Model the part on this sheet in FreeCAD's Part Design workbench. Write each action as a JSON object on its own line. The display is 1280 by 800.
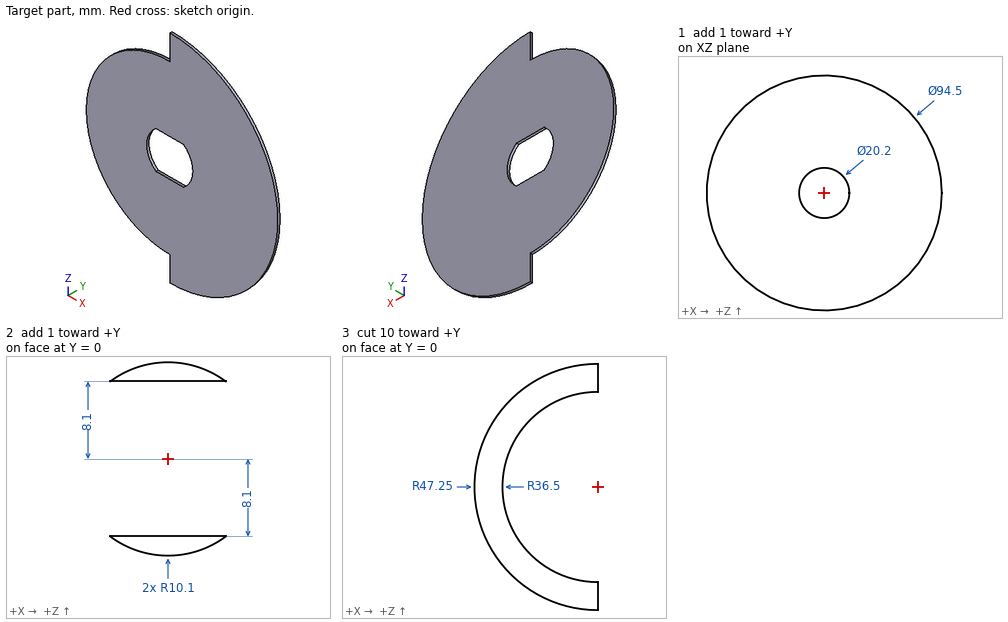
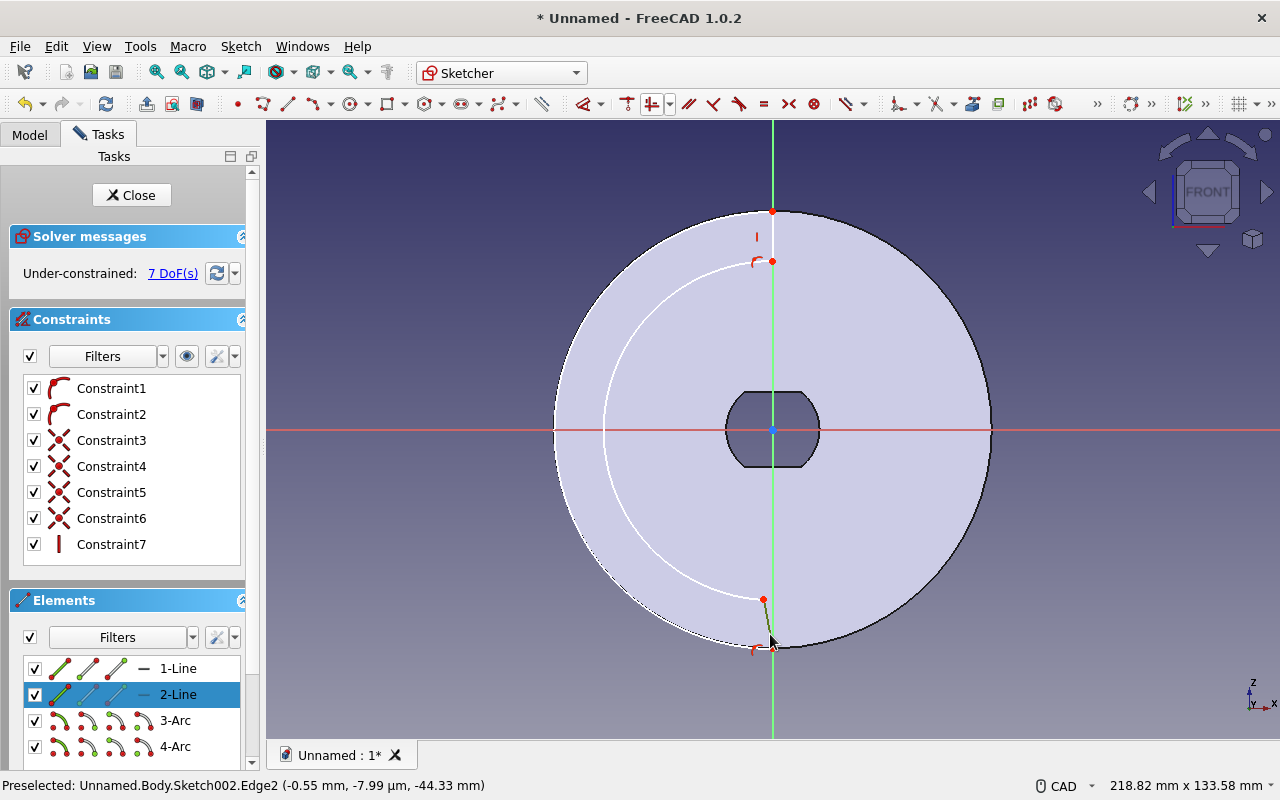
{"action": "left_click", "coordinate": [670, 104]}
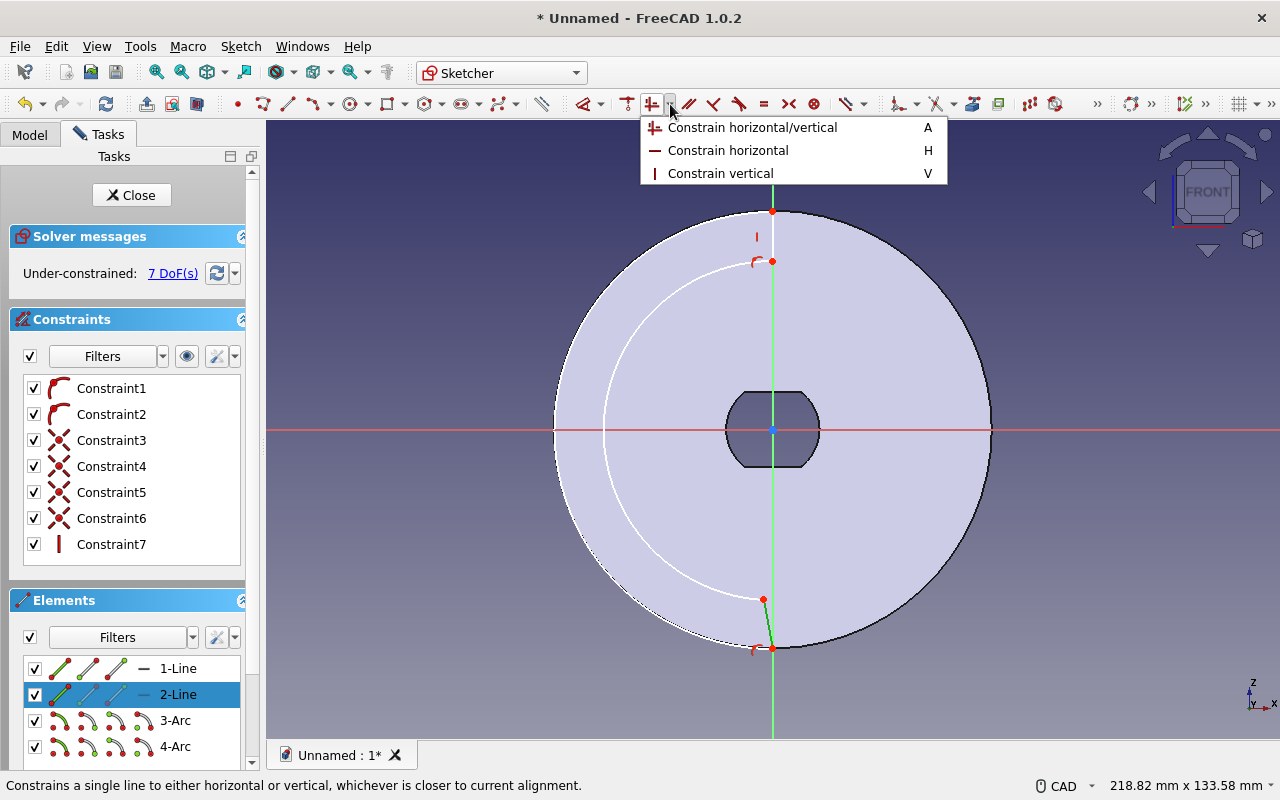
{"action": "left_click", "coordinate": [794, 174]}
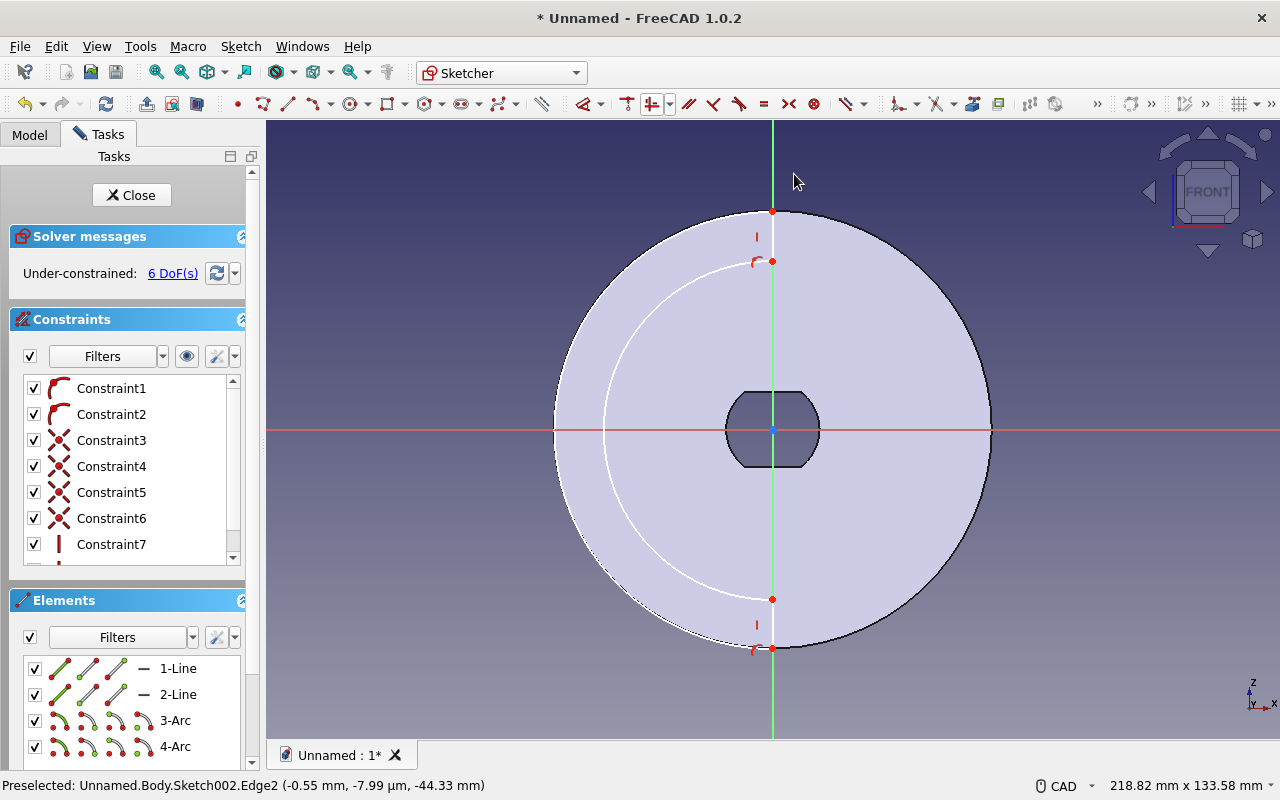
{"action": "left_click", "coordinate": [596, 302]}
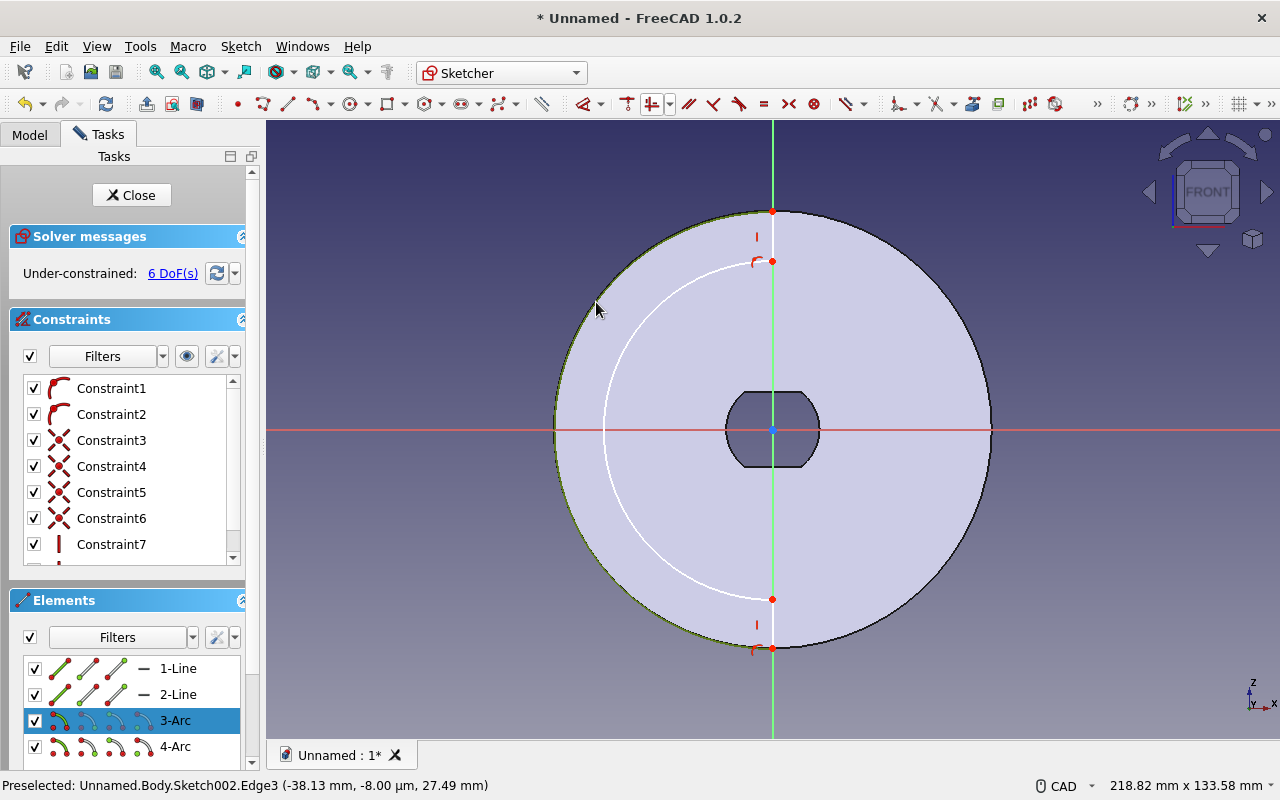
{"action": "left_click", "coordinate": [636, 331]}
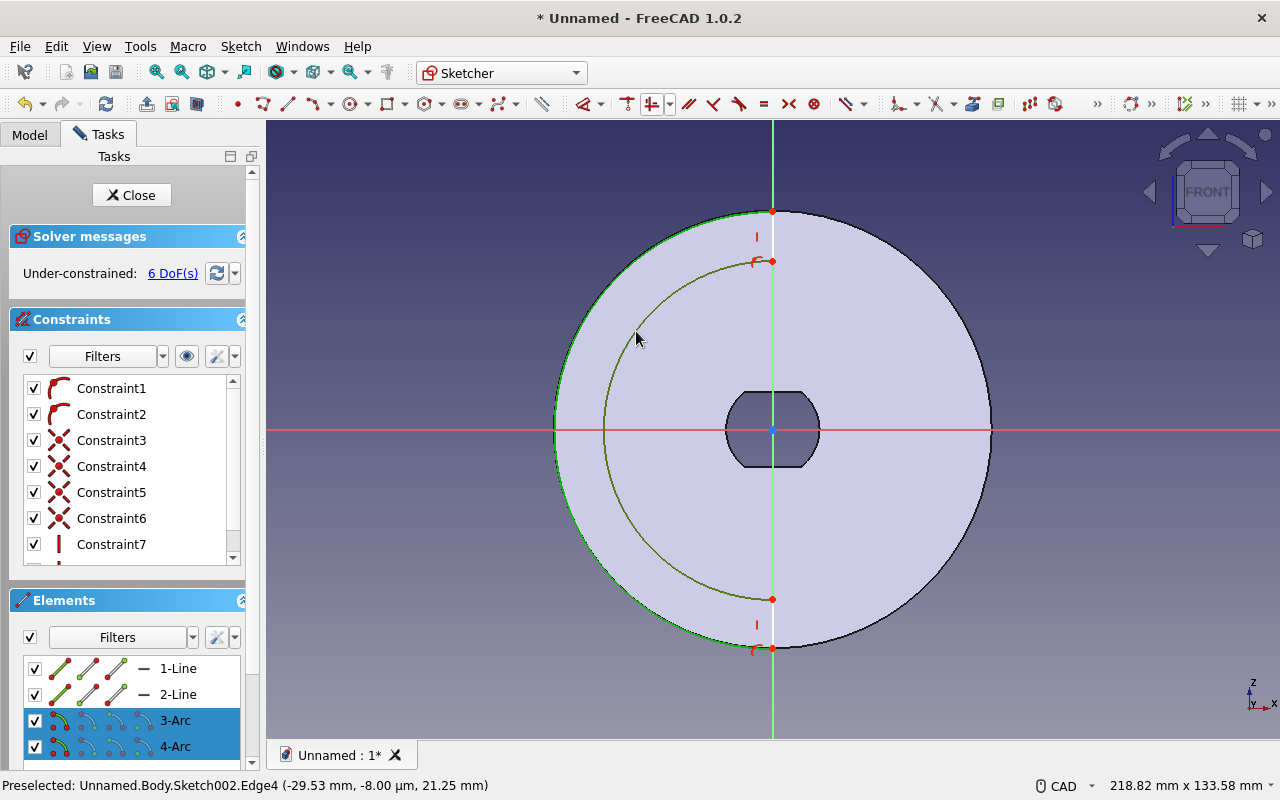
{"action": "left_click", "coordinate": [627, 104]}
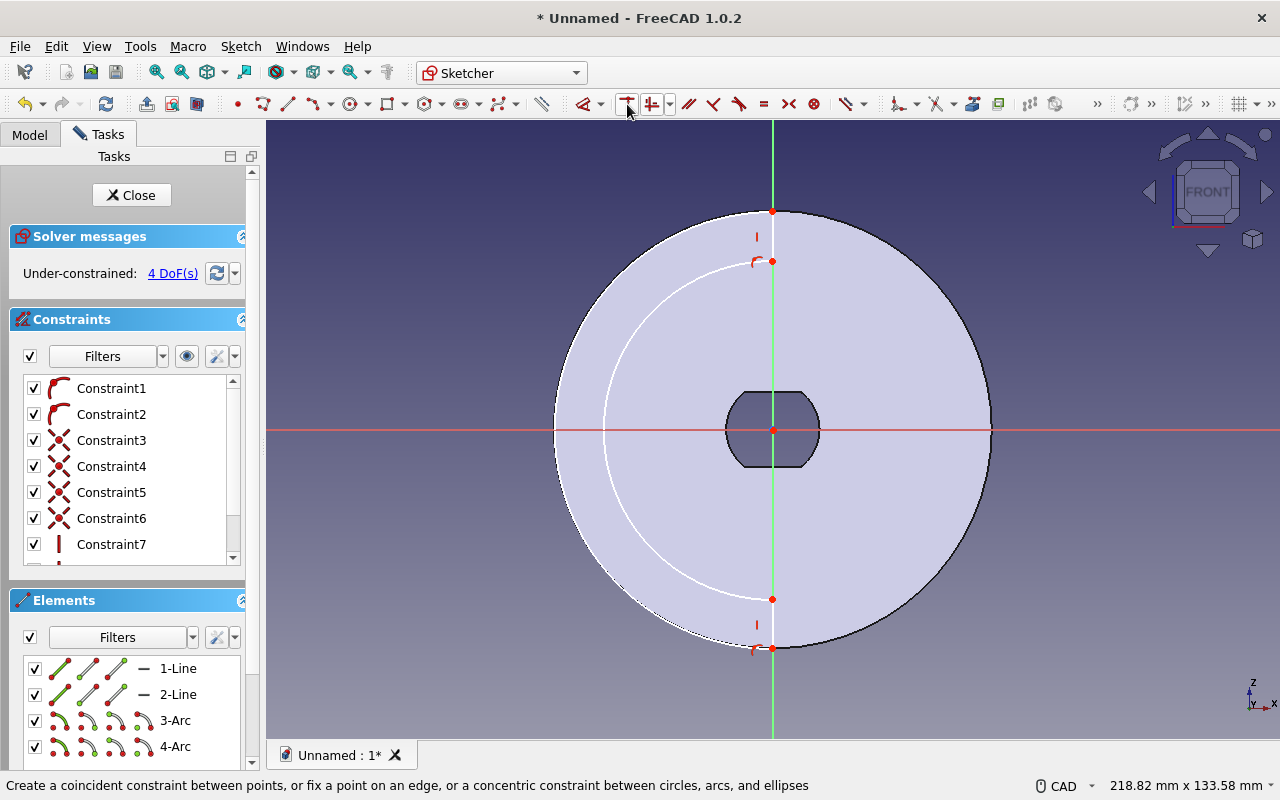
{"action": "left_click_drag", "start_coordinate": [763, 420], "coordinate": [783, 441]}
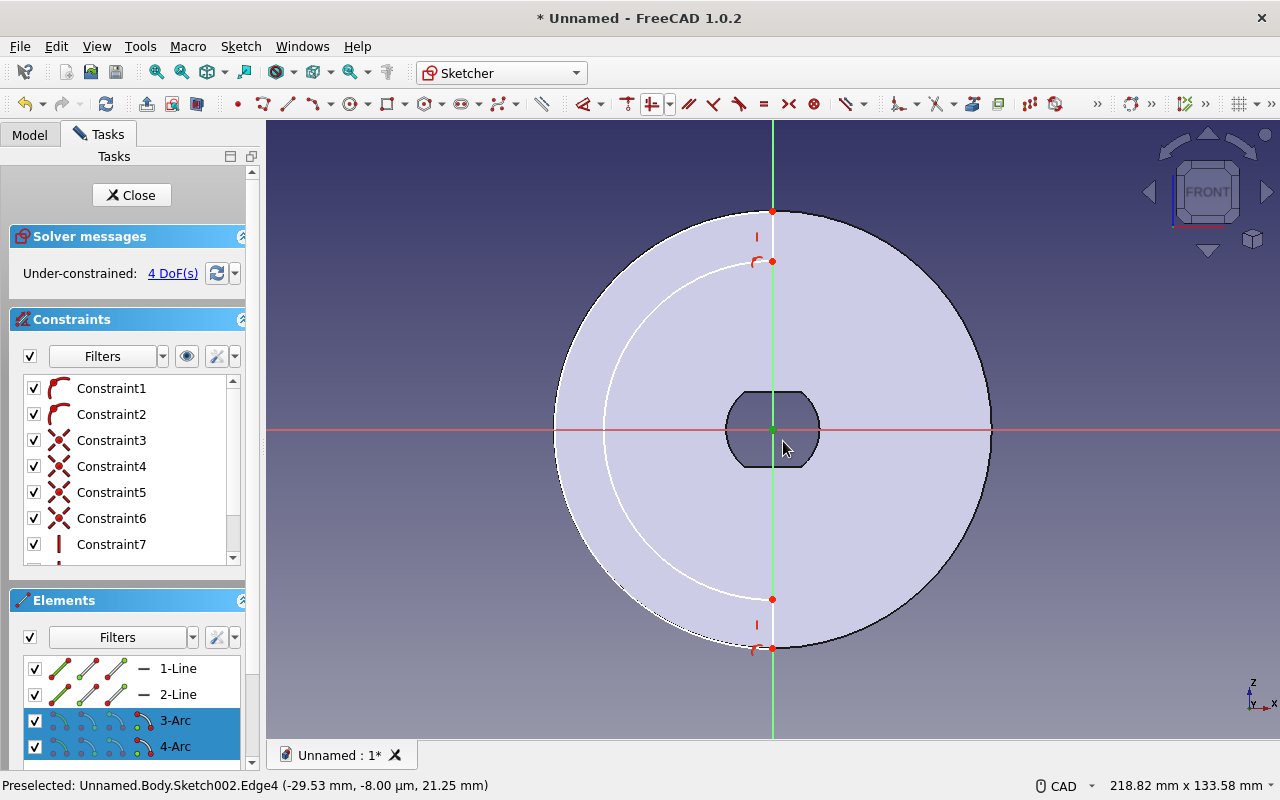
{"action": "left_click", "coordinate": [627, 104]}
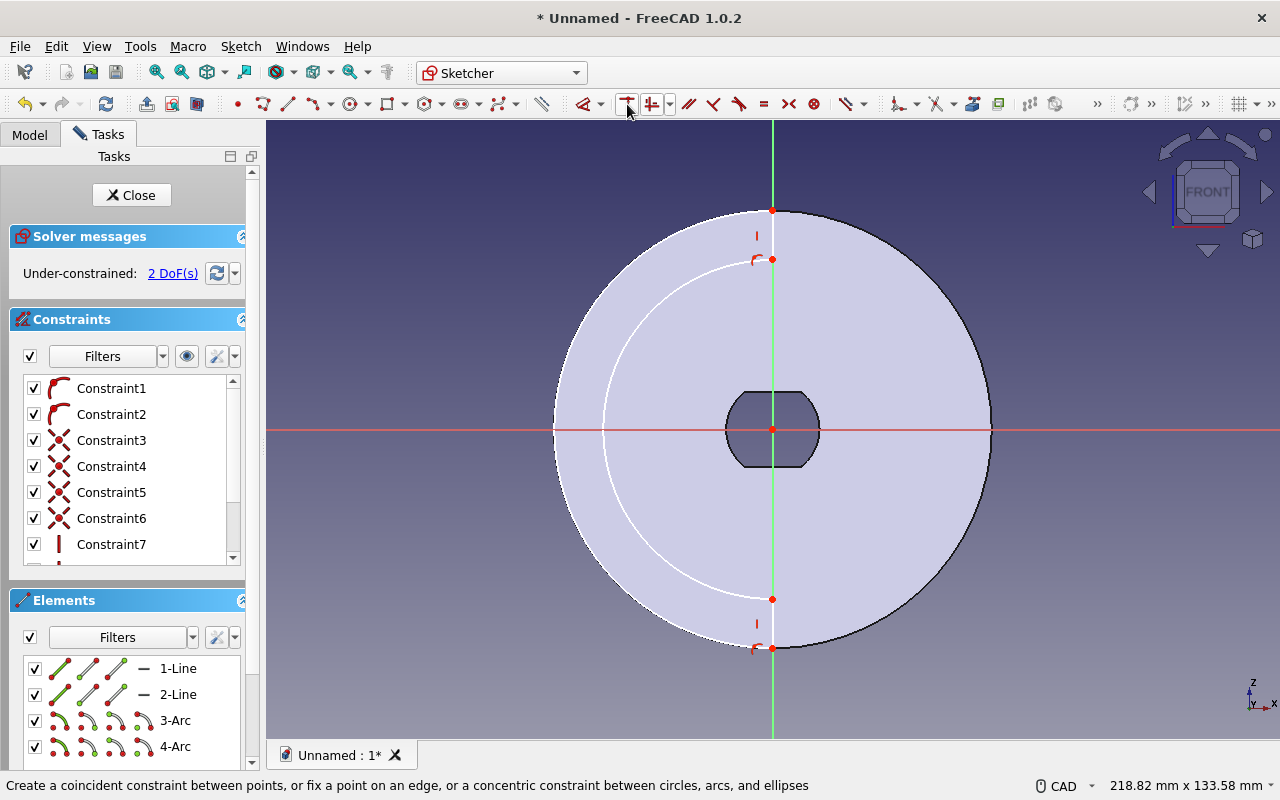
{"action": "left_click", "coordinate": [582, 104]}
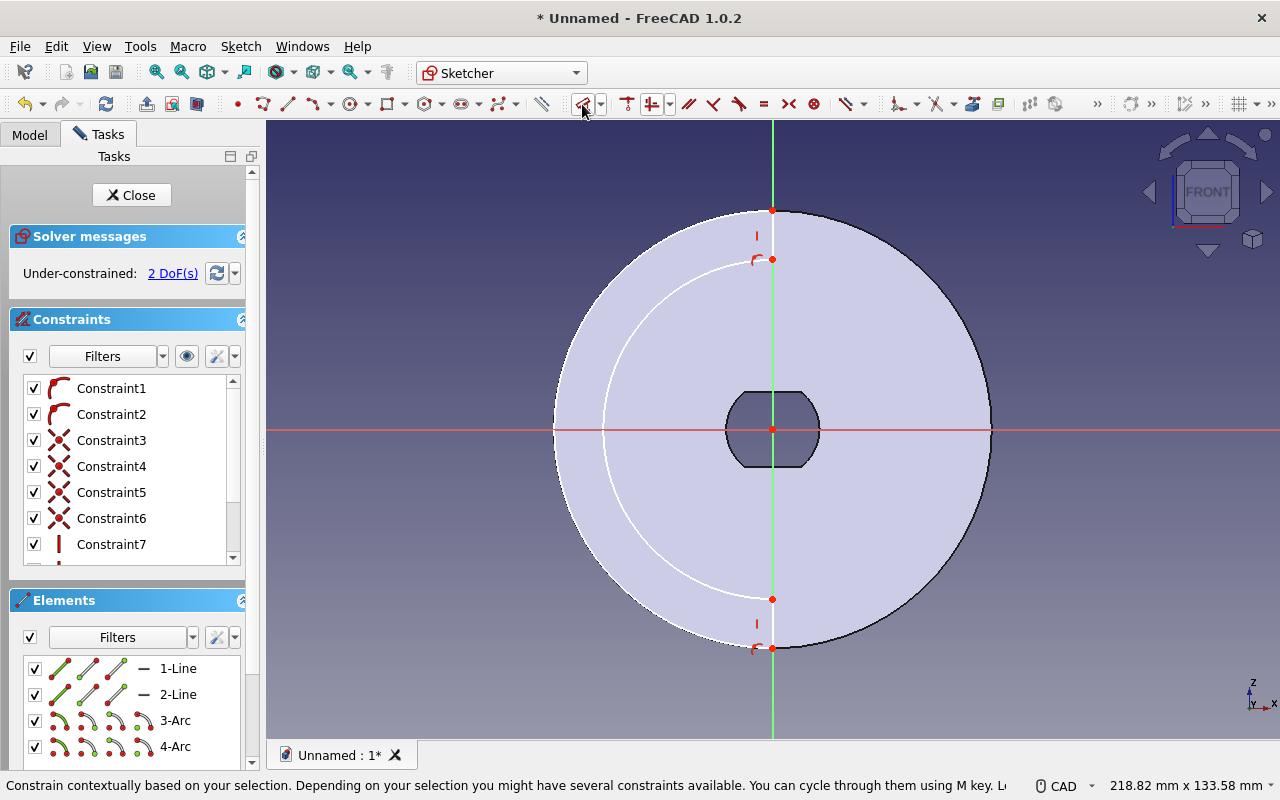
{"action": "left_click", "coordinate": [596, 301]}
{"action": "left_click", "coordinate": [570, 282]}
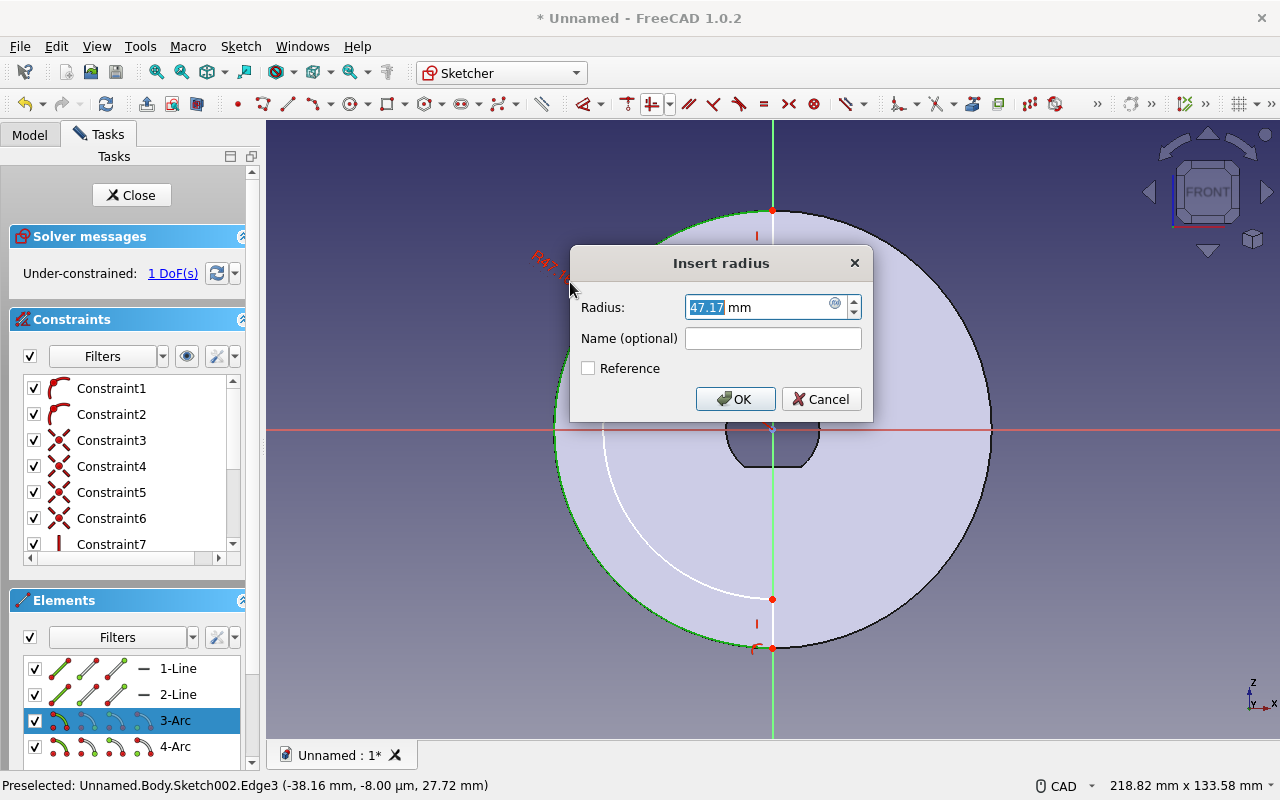
{"action": "type", "text": "47.25"}
{"action": "key", "text": "Return"}